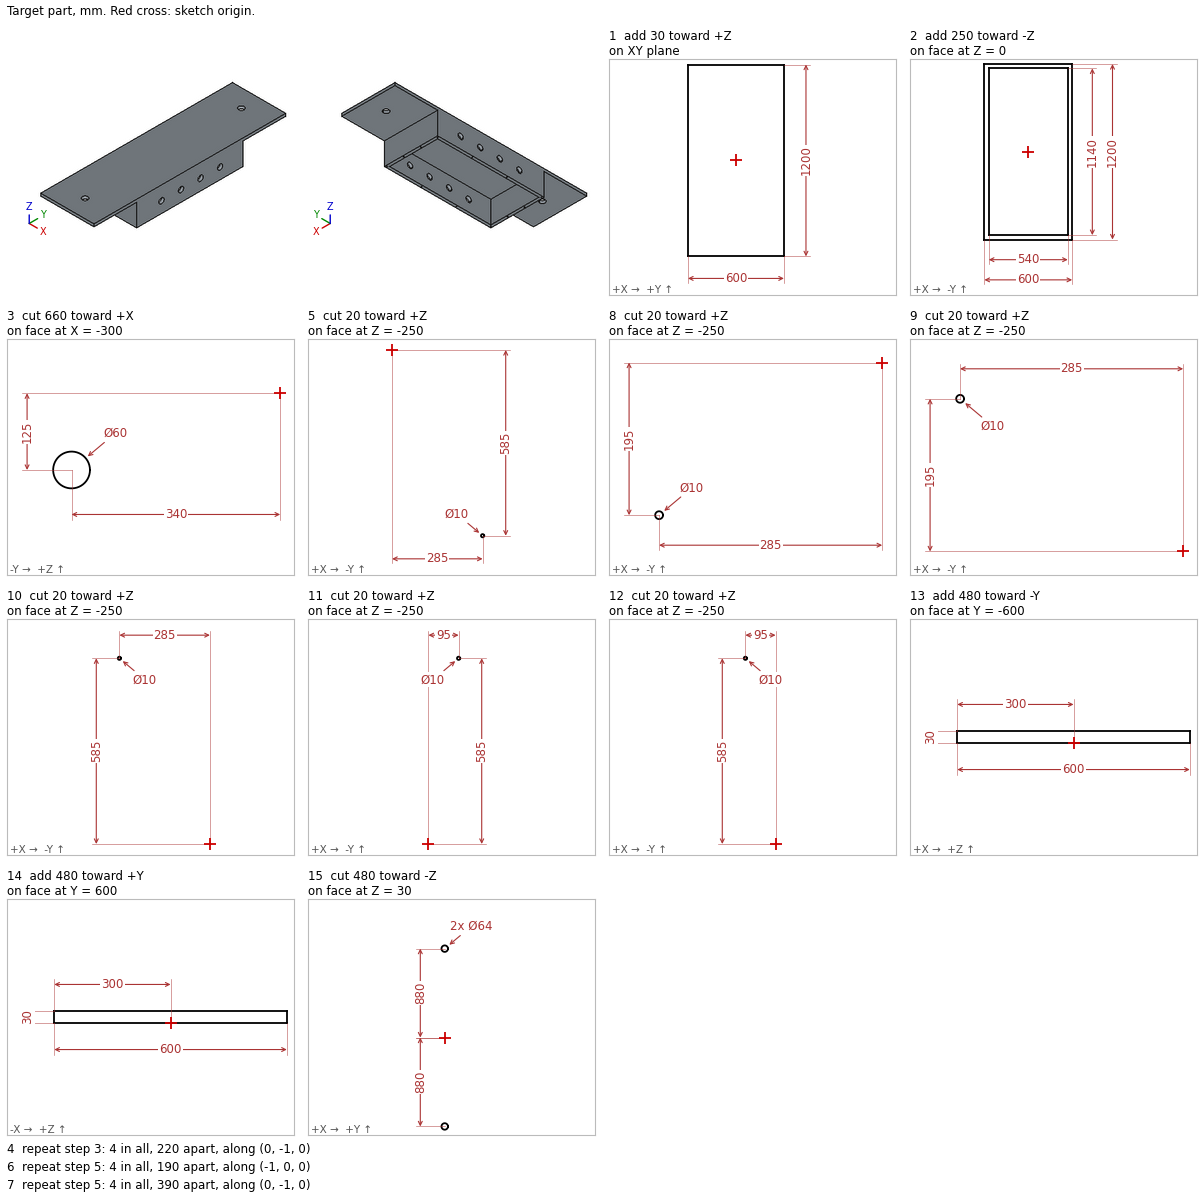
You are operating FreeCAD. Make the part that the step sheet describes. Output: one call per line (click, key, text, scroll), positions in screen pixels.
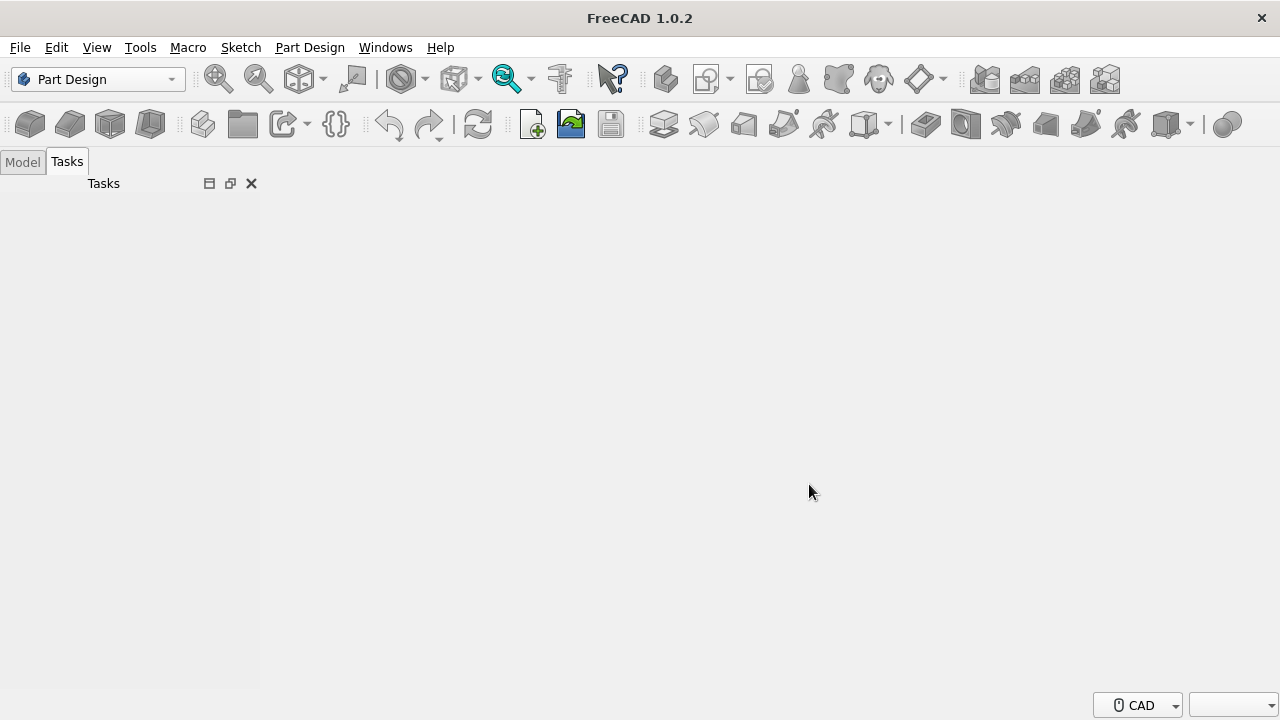
click(532, 124)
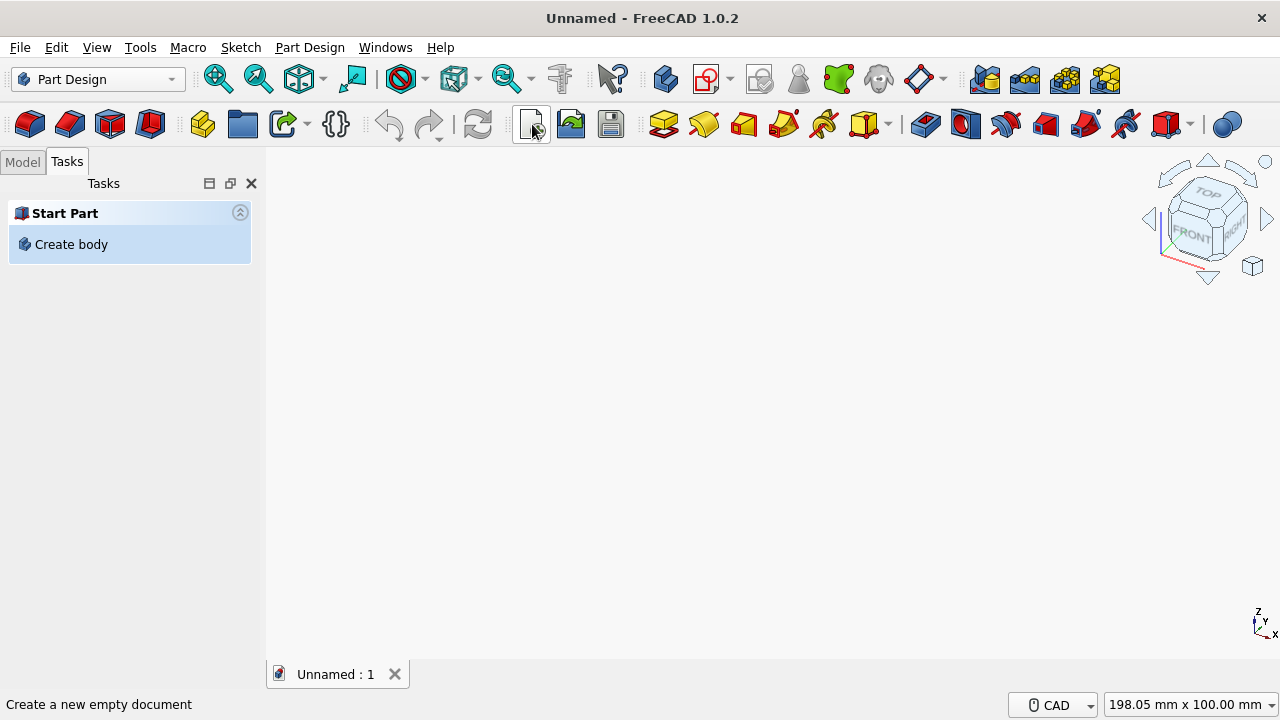
click(706, 80)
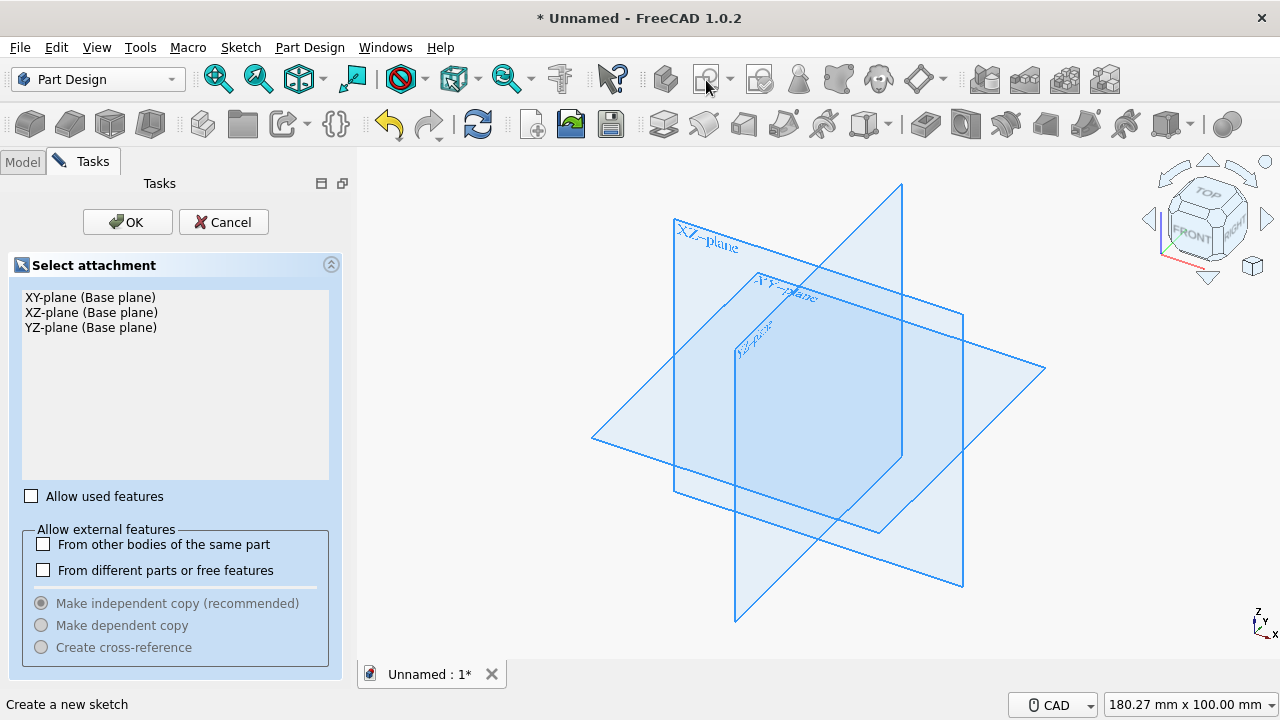
click(82, 298)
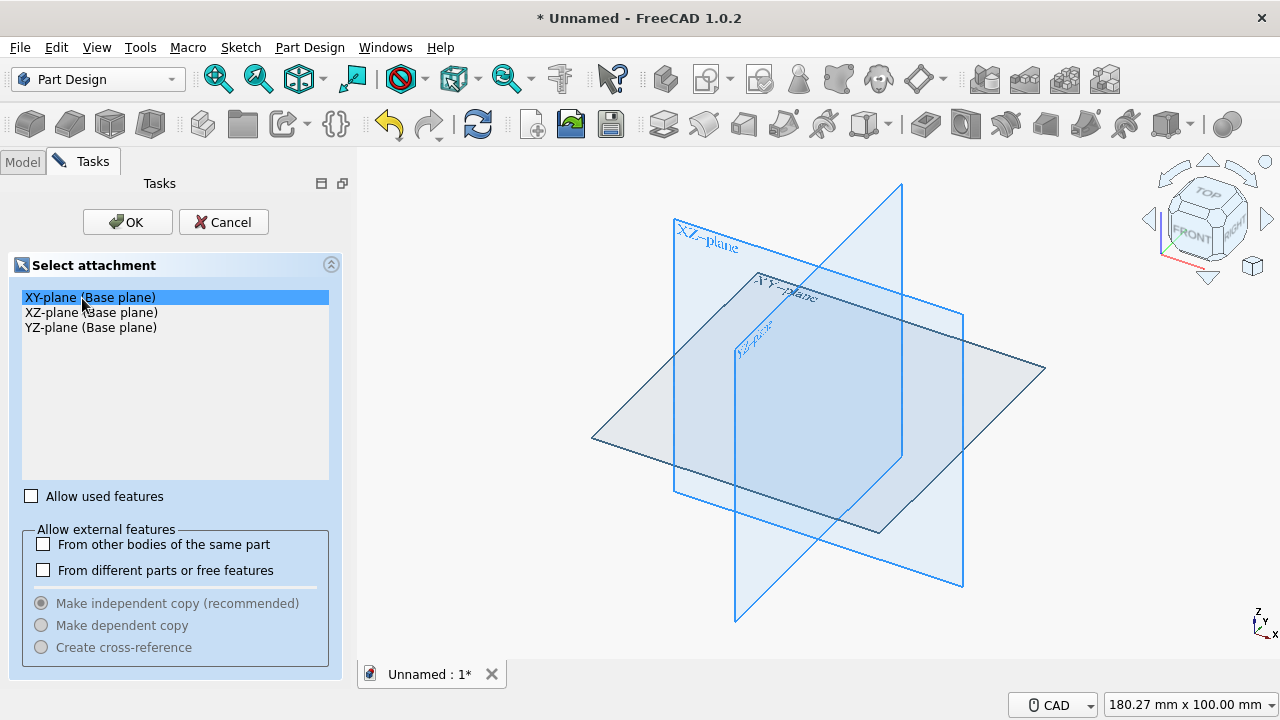
click(128, 222)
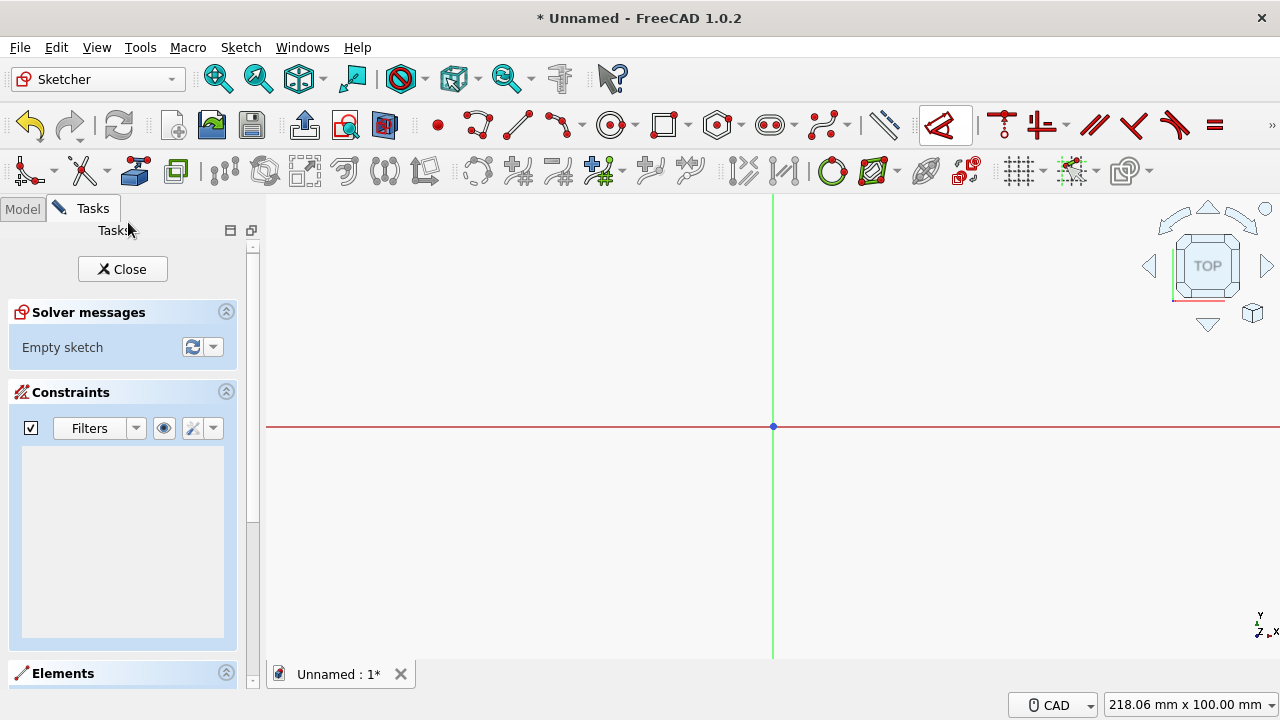
scroll(701, 426, down, 15)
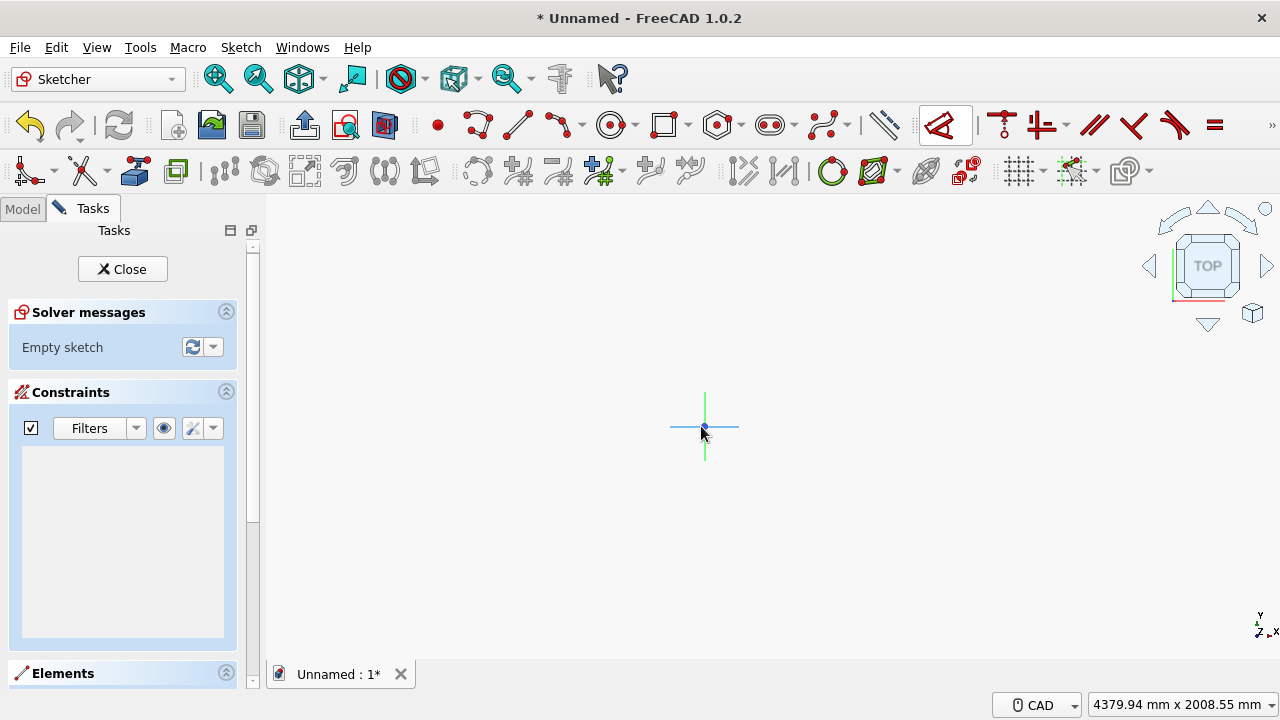
click(690, 126)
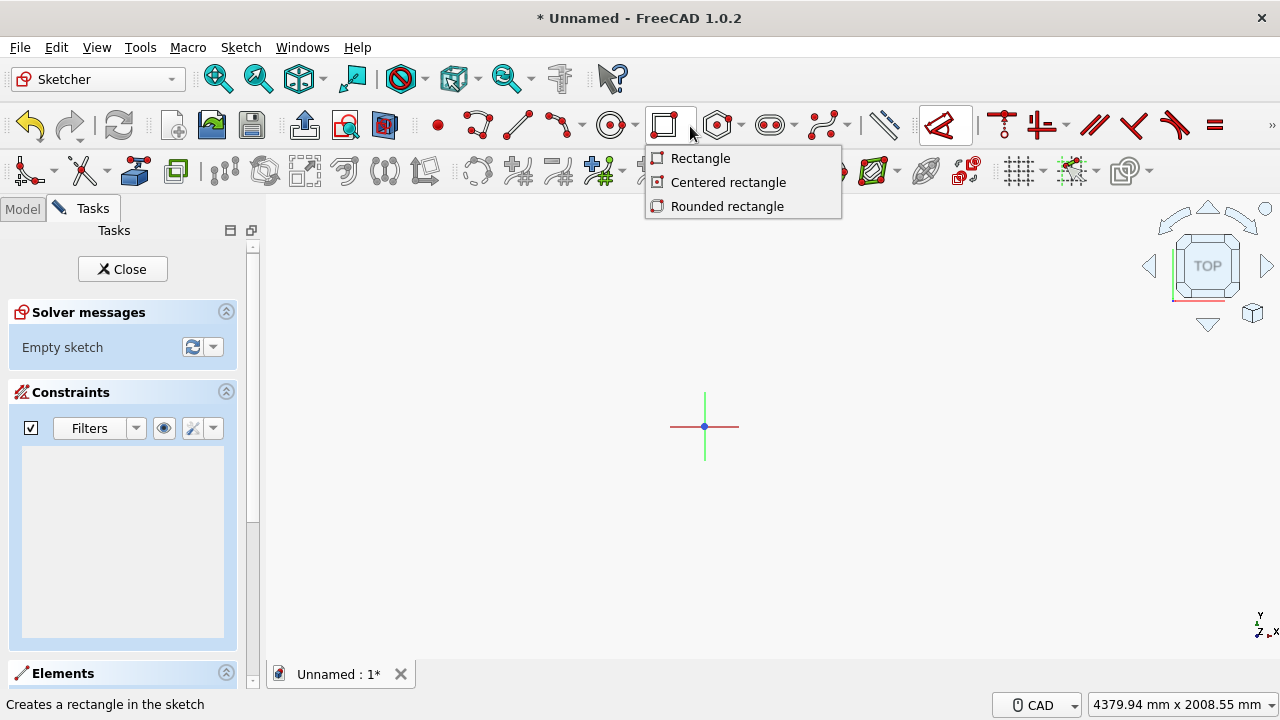
click(744, 182)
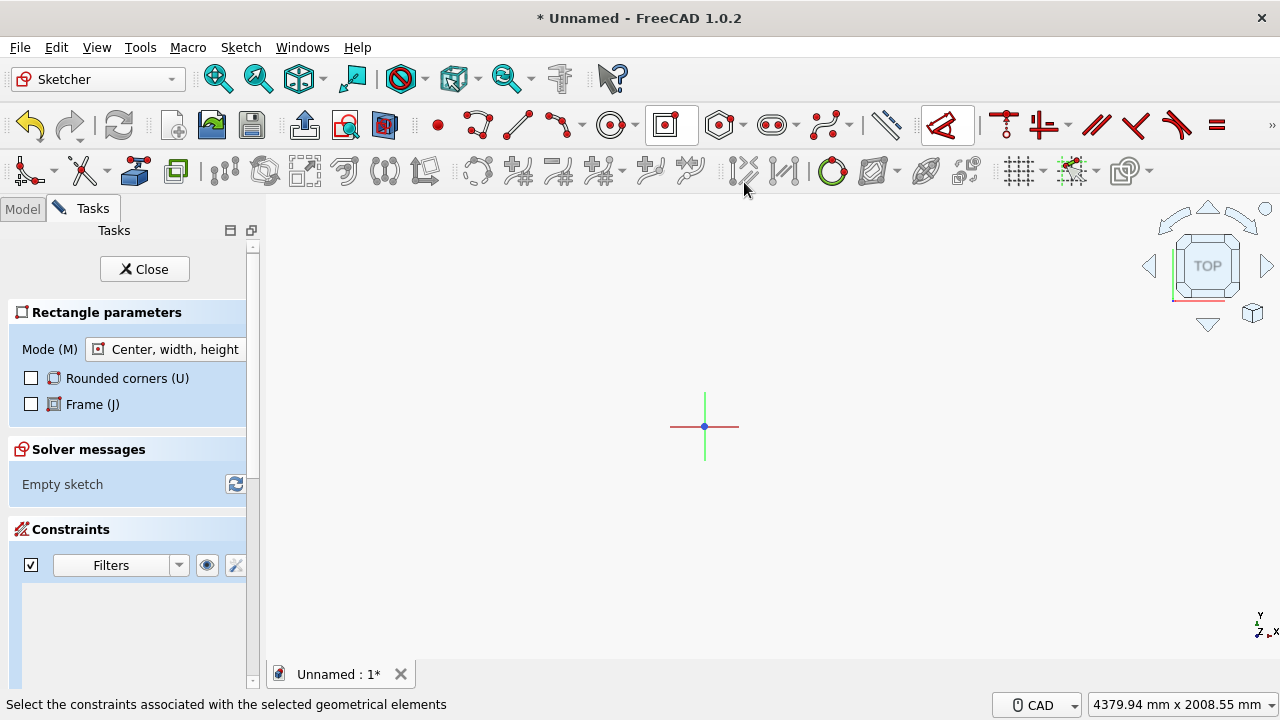
click(705, 426)
move(774, 288)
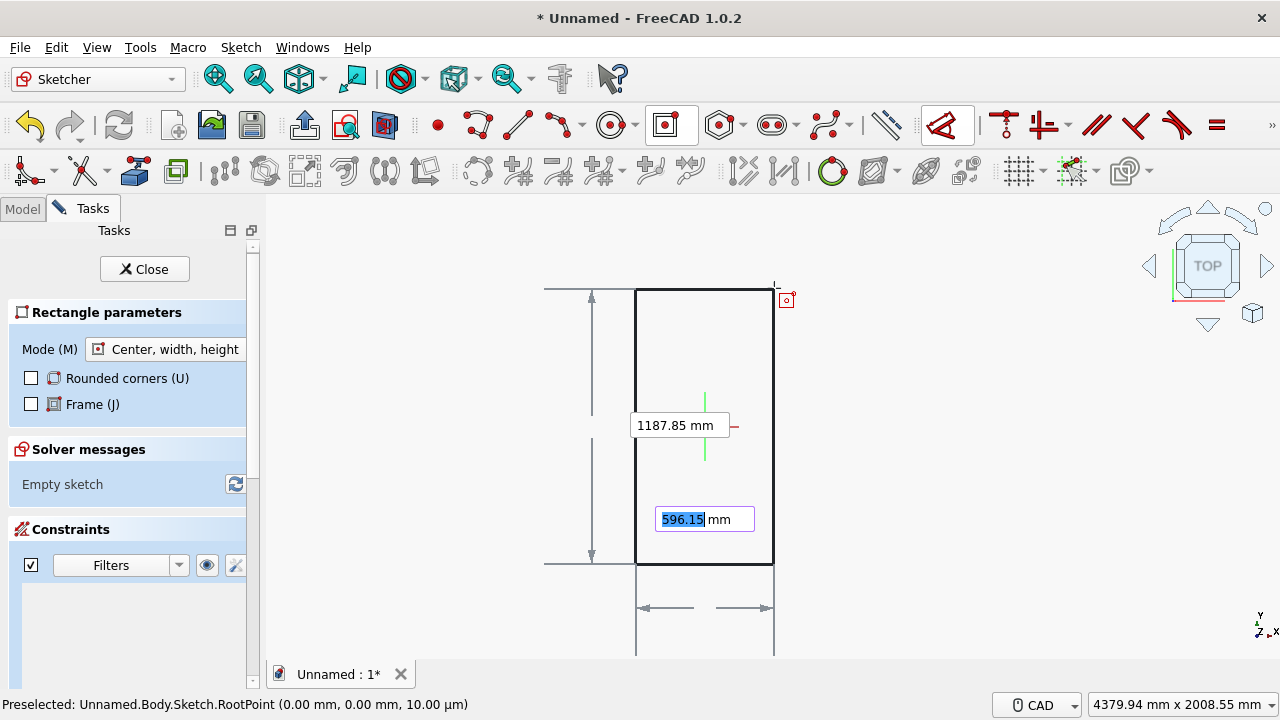
text(600)
key(Tab)
text(1200)
key(Return)
key(Escape)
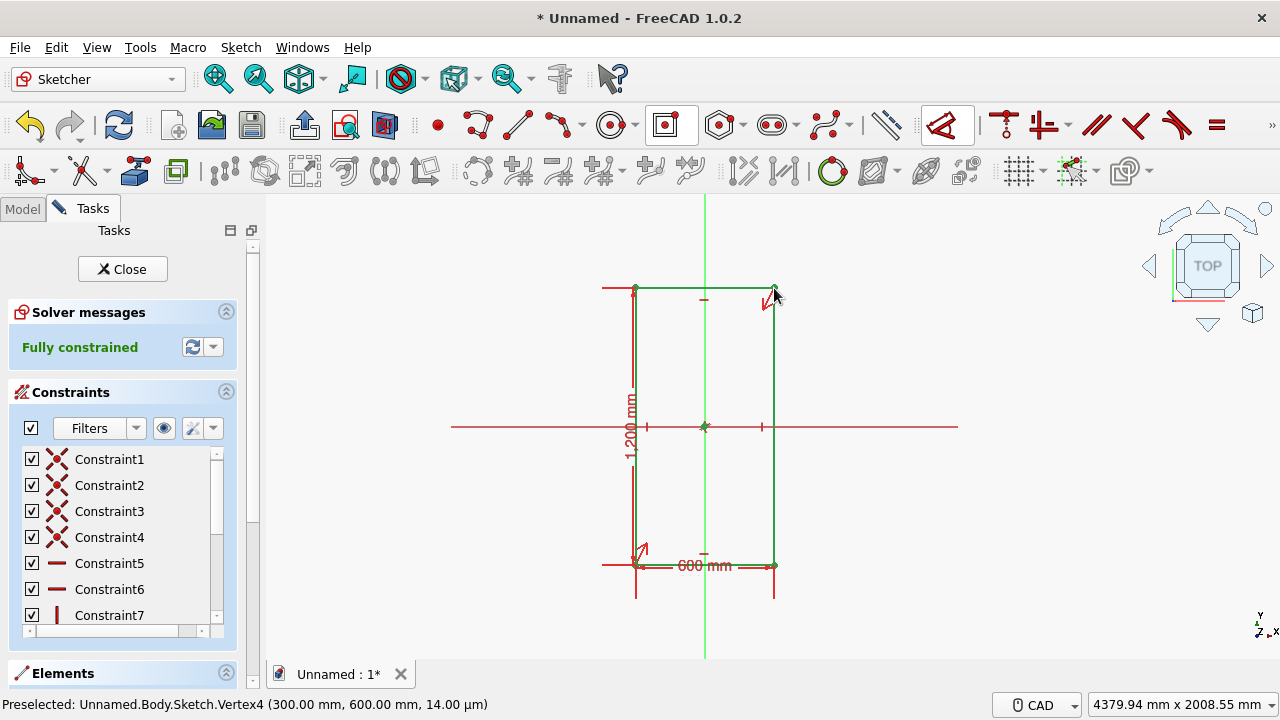
click(123, 269)